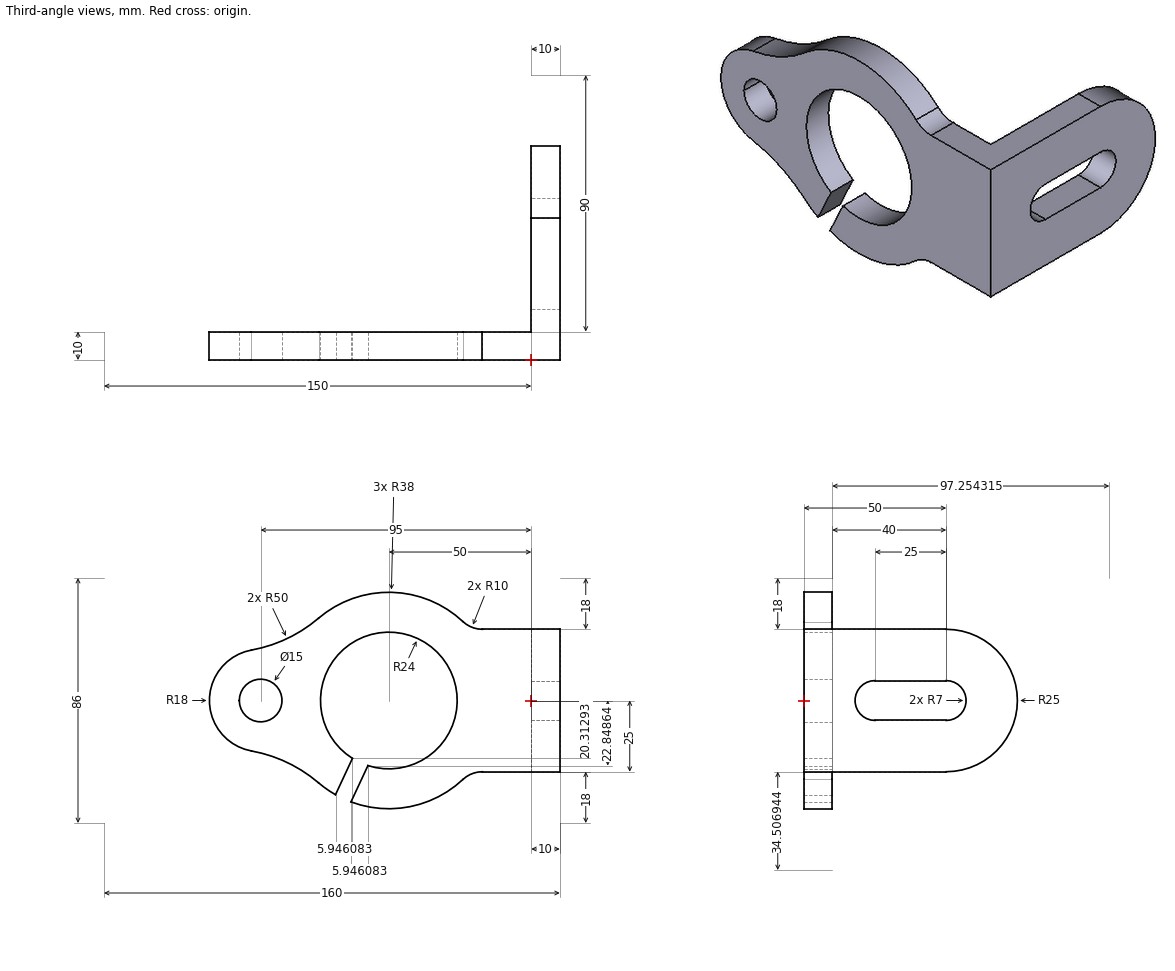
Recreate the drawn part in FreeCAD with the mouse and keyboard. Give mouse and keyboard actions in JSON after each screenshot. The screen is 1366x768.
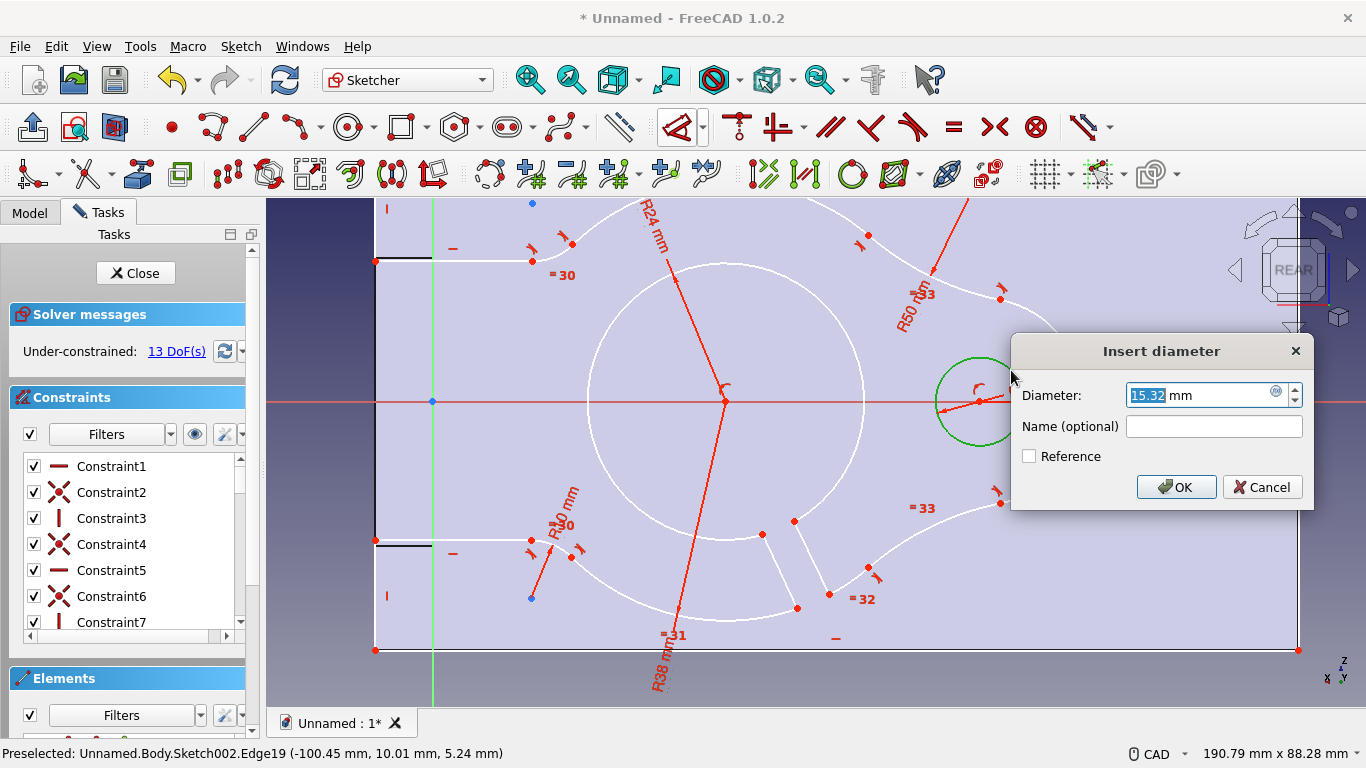
{"action": "type", "text": "15"}
{"action": "key", "text": "Return"}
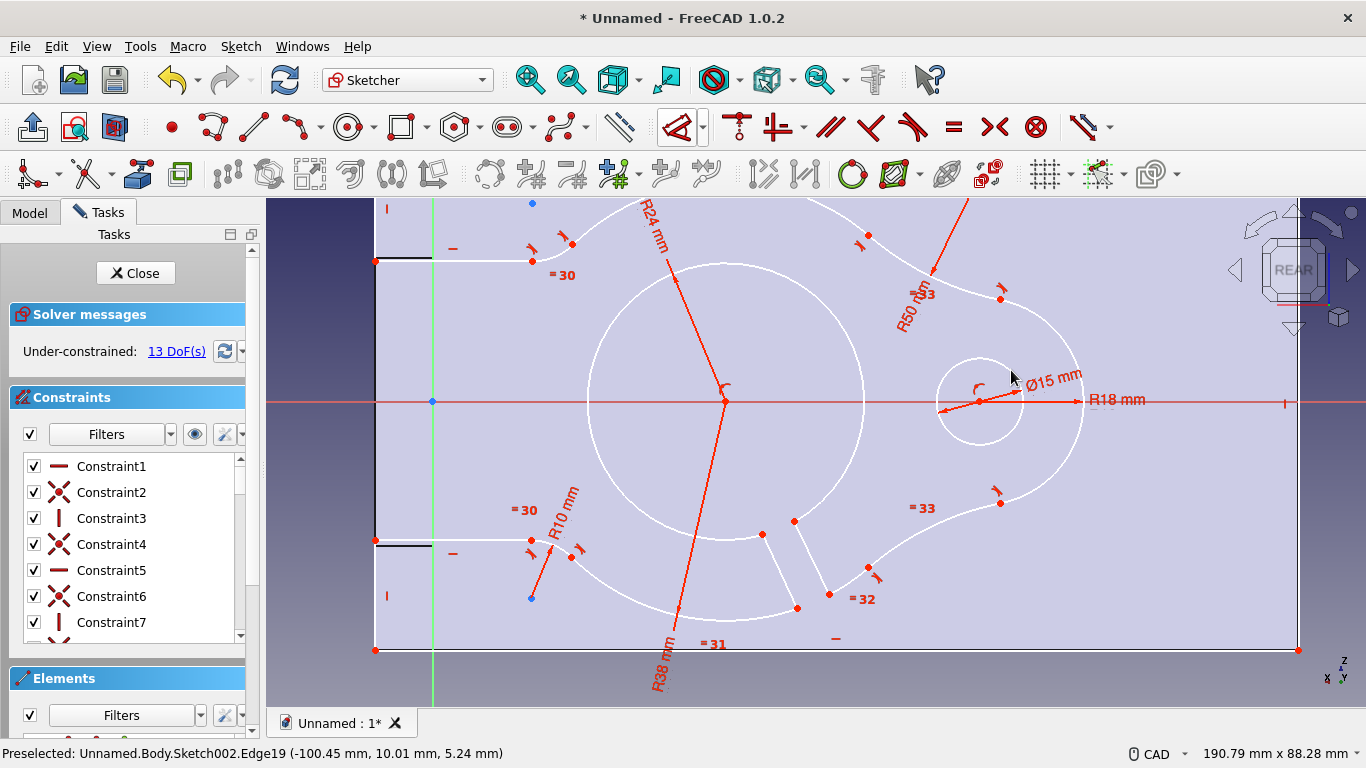
{"action": "left_click", "coordinate": [375, 574]}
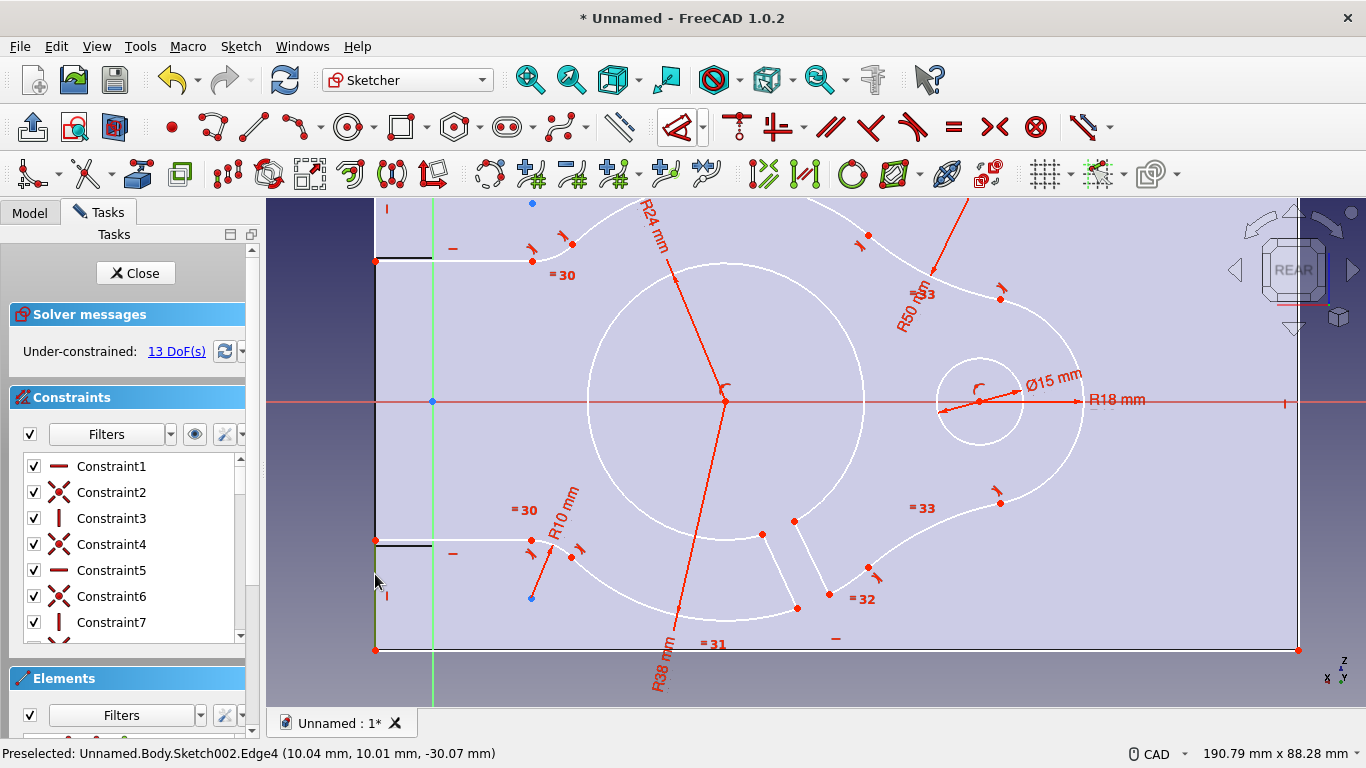
{"action": "left_click", "coordinate": [702, 128]}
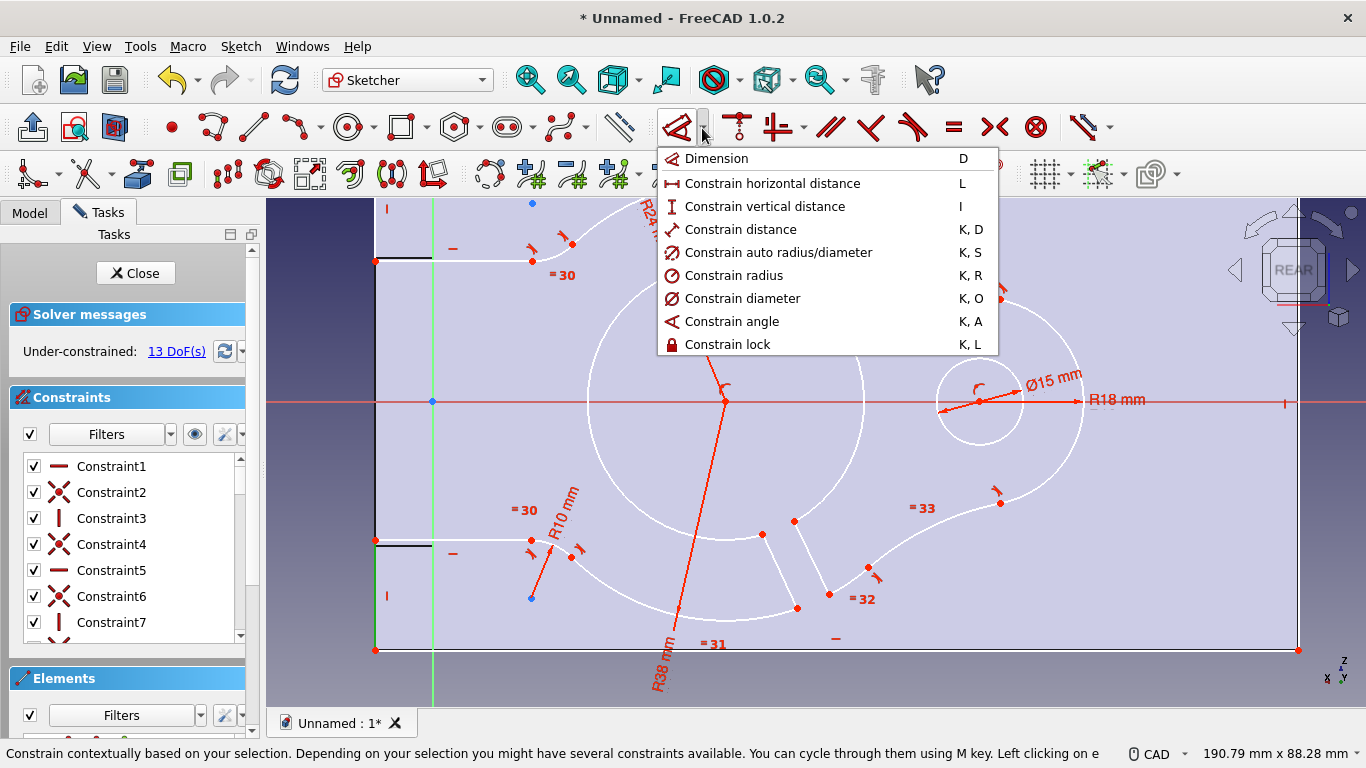
{"action": "left_click", "coordinate": [828, 206]}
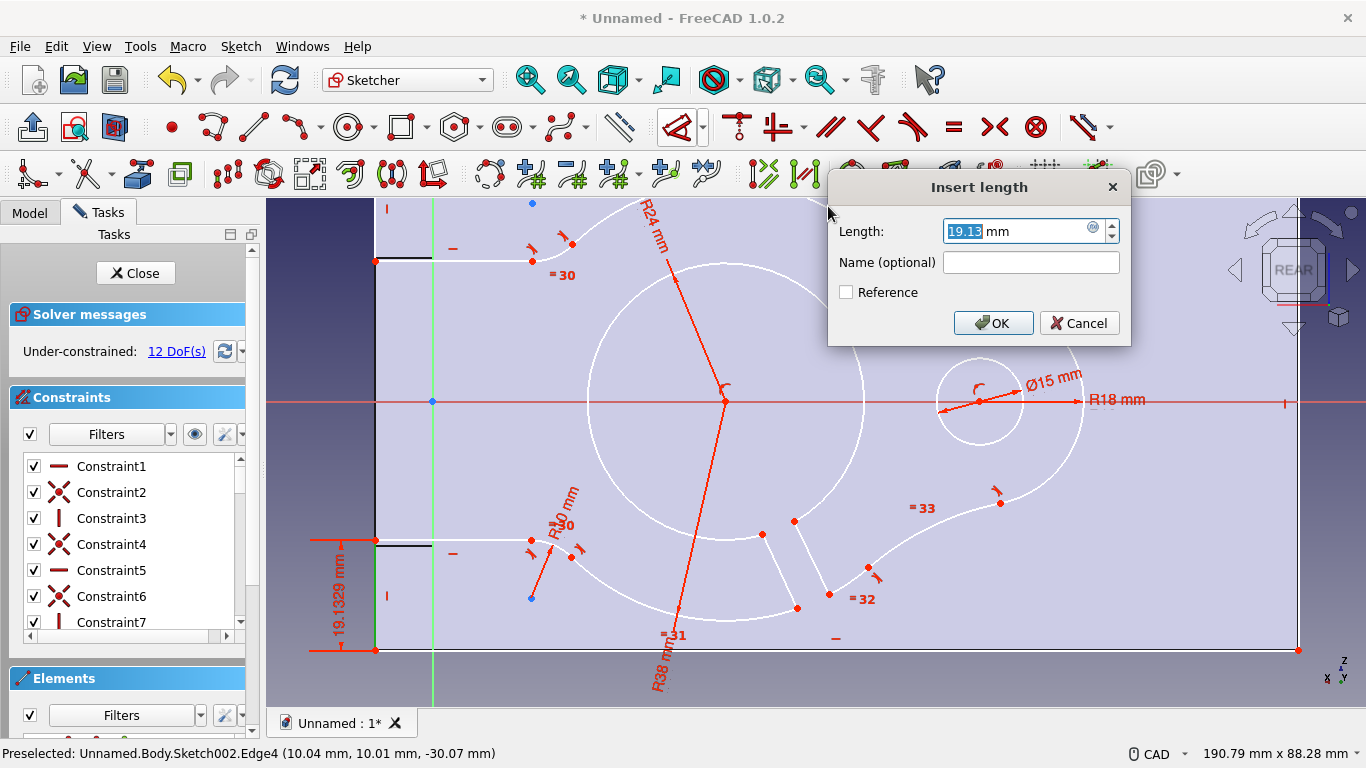
{"action": "type", "text": "18"}
{"action": "key", "text": "Return"}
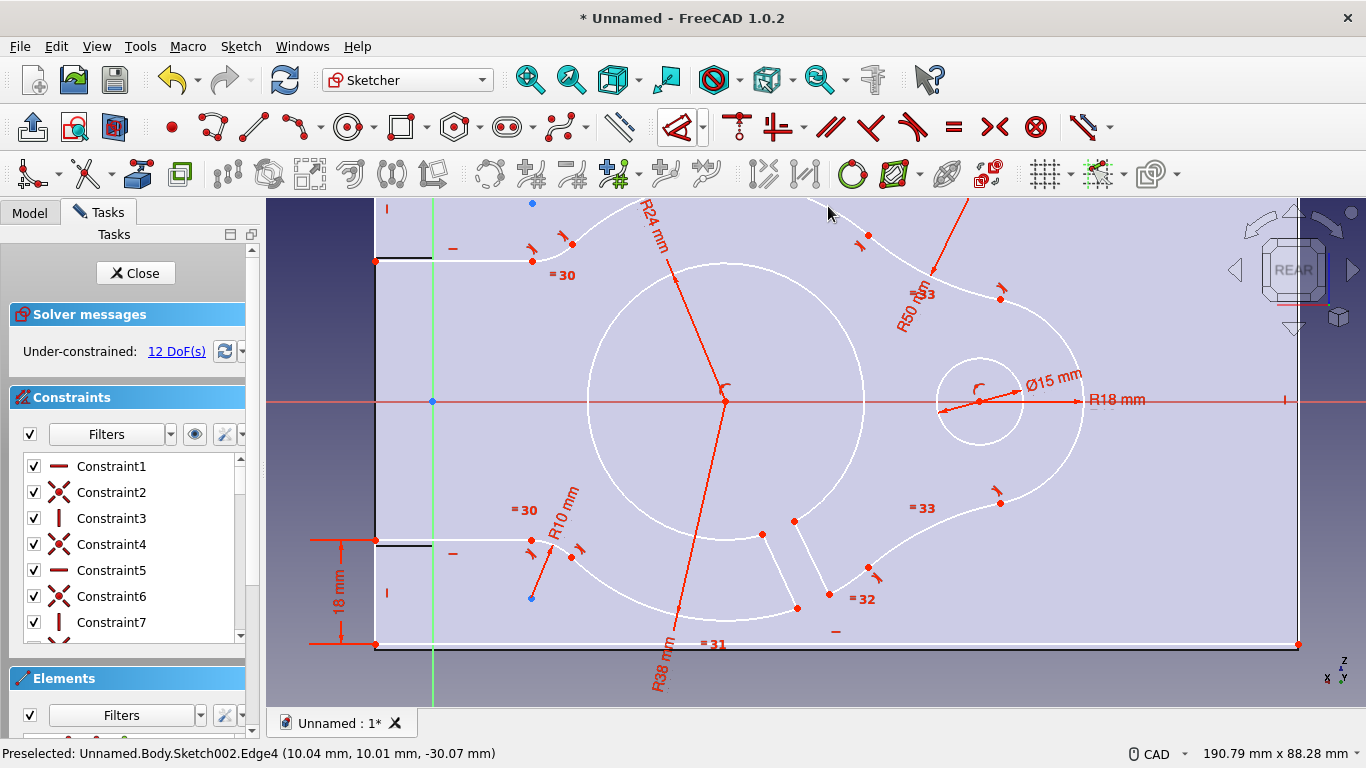
{"action": "scroll", "coordinate": [566, 556], "scroll_direction": "down", "scroll_amount": 2}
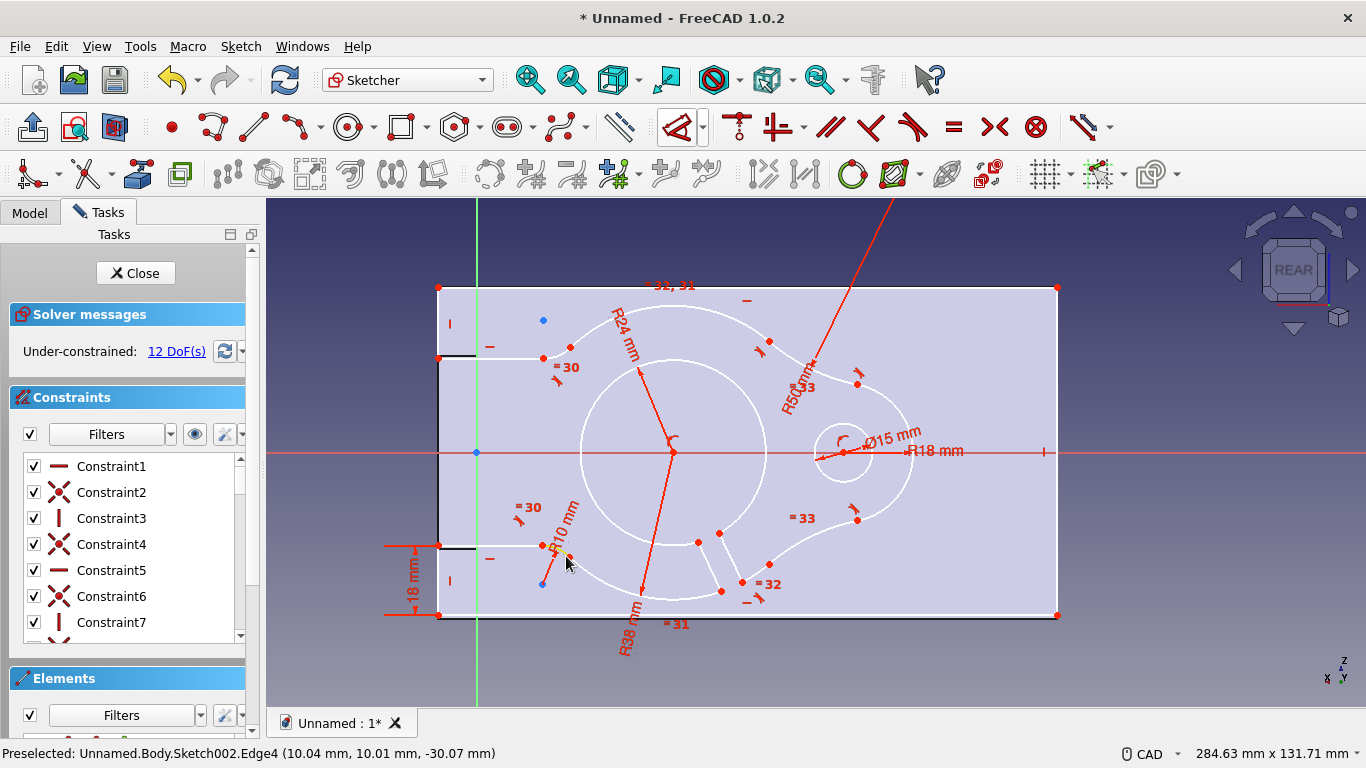
{"action": "left_click", "coordinate": [1057, 517]}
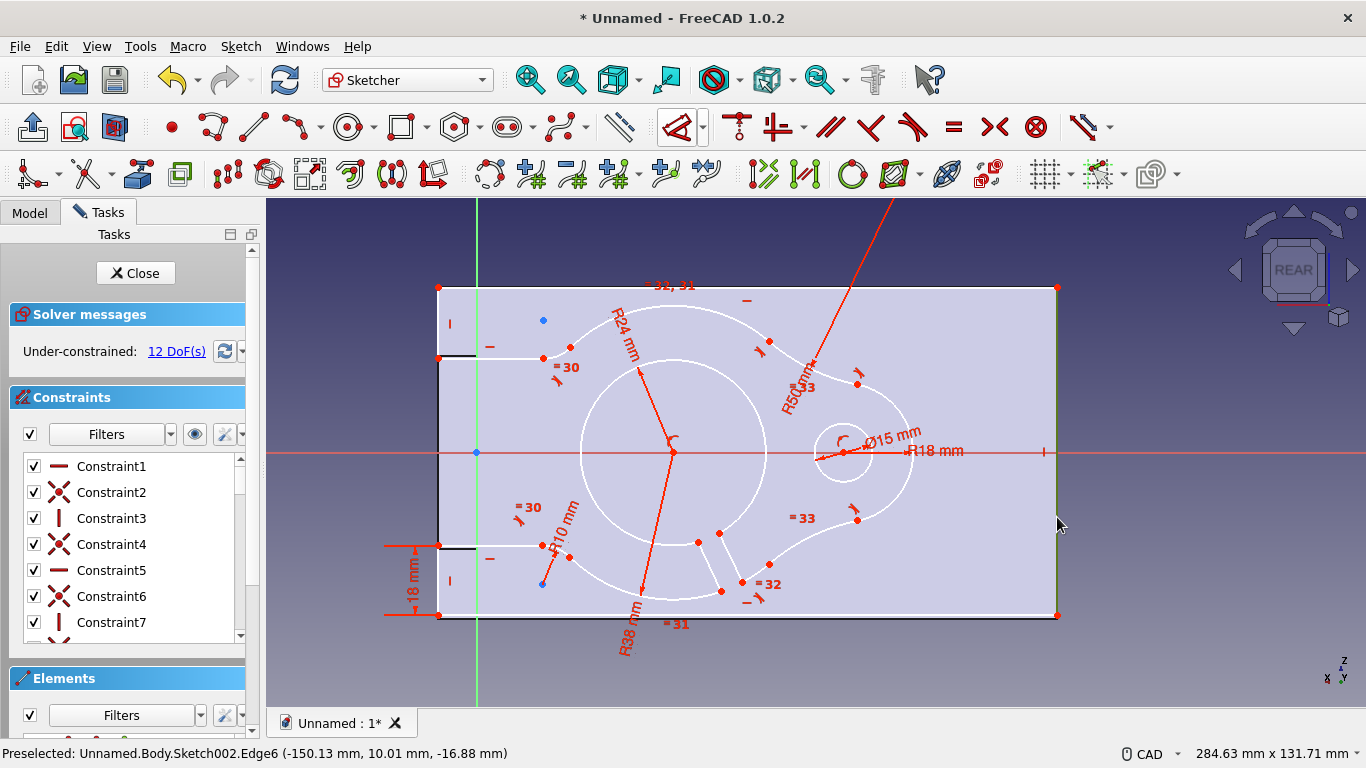
{"action": "key", "text": "i"}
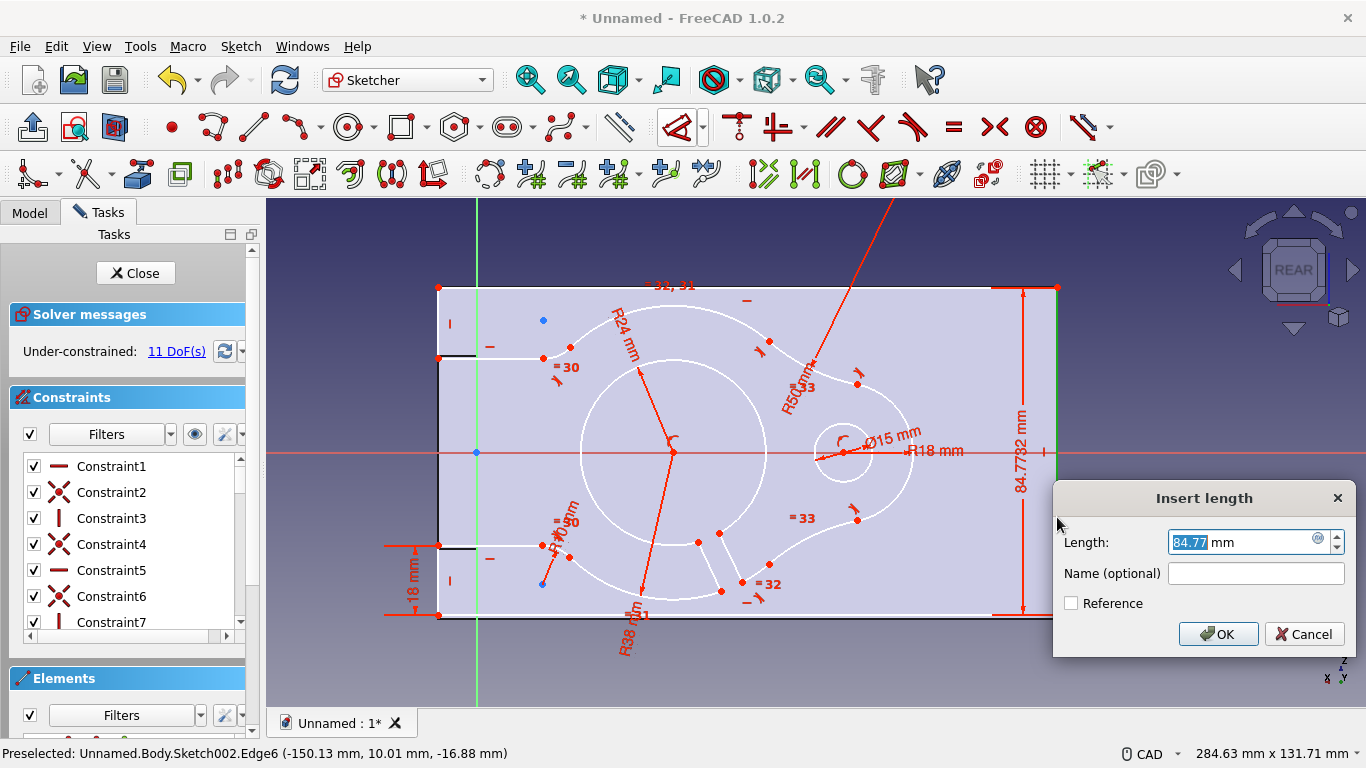
{"action": "type", "text": "86"}
{"action": "key", "text": "Return"}